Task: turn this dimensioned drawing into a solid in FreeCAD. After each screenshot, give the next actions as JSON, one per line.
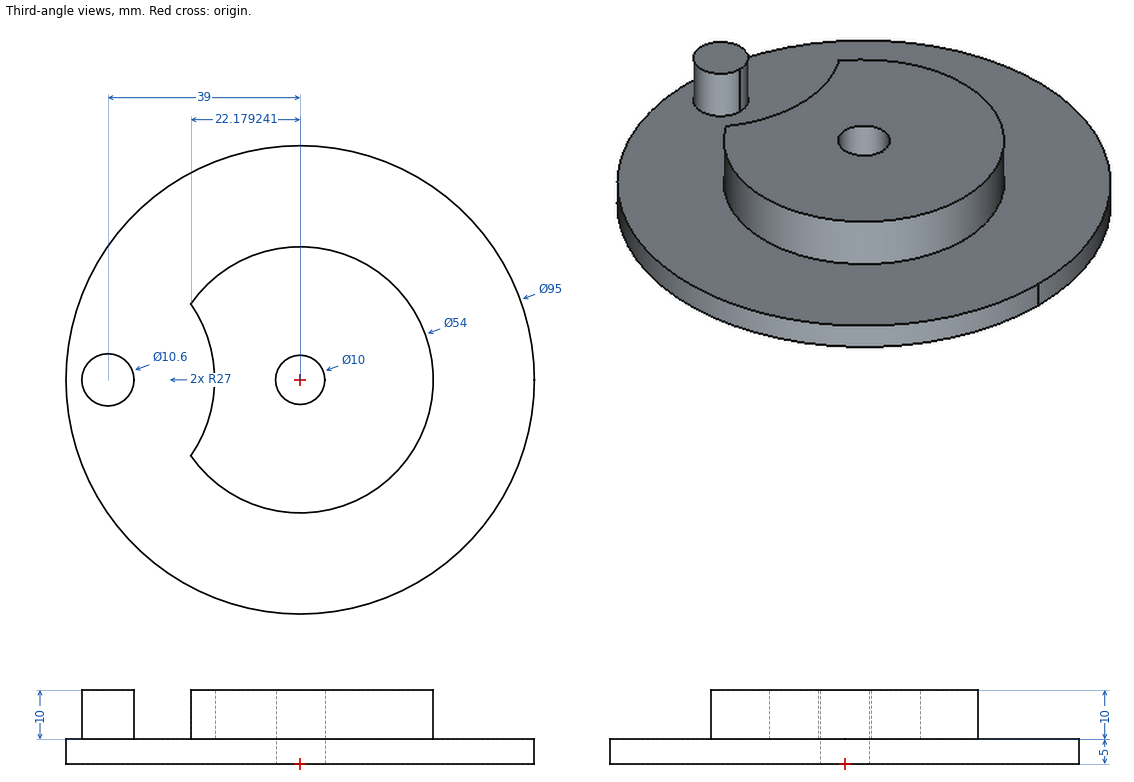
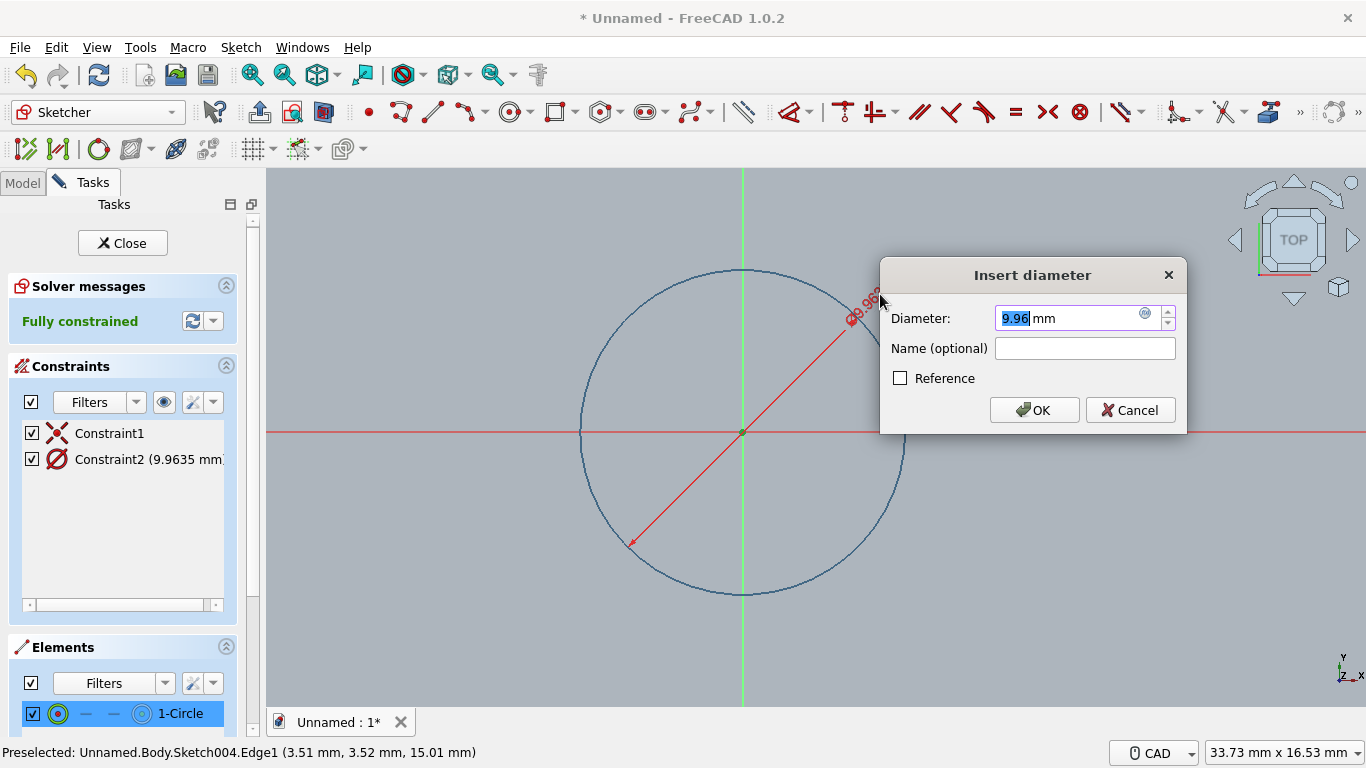
{"action": "type", "text": "10"}
{"action": "key", "text": "Return"}
{"action": "key", "text": "Escape"}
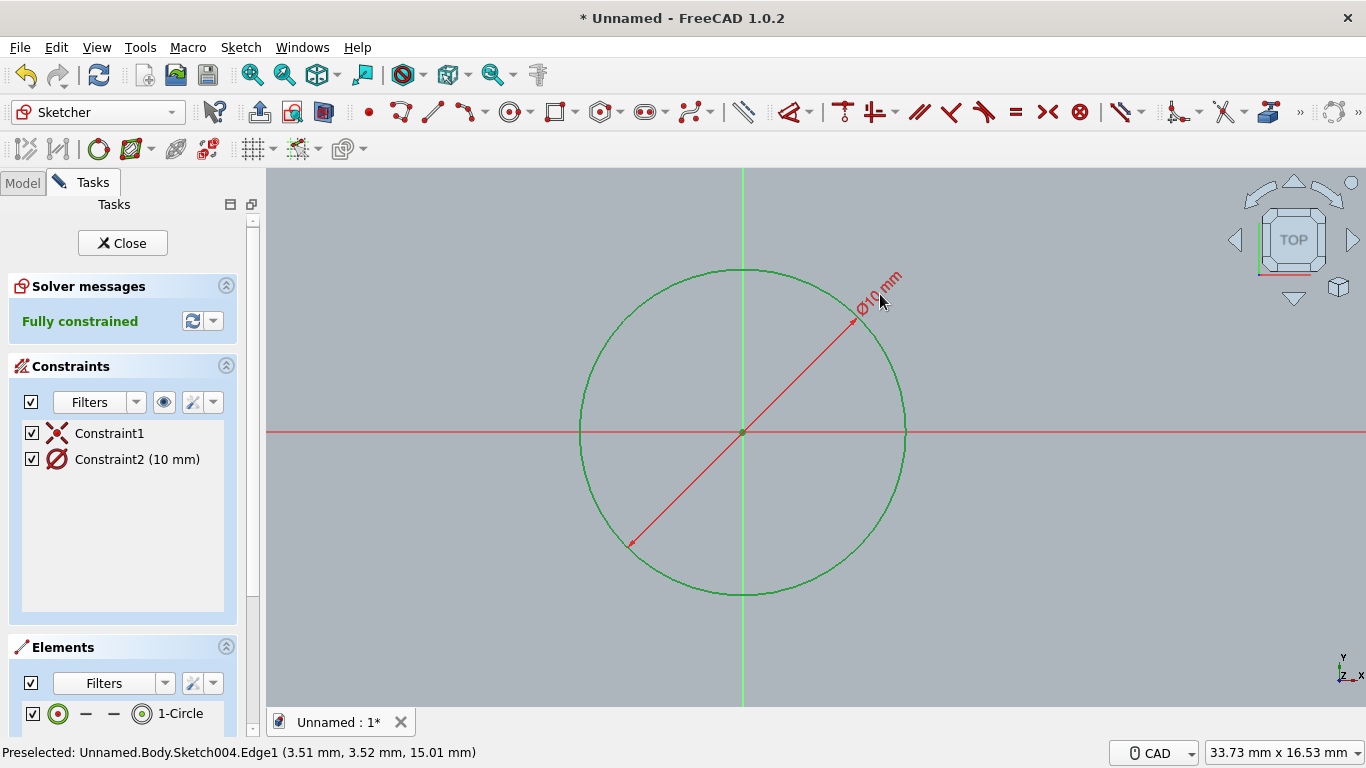
{"action": "left_click", "coordinate": [123, 243]}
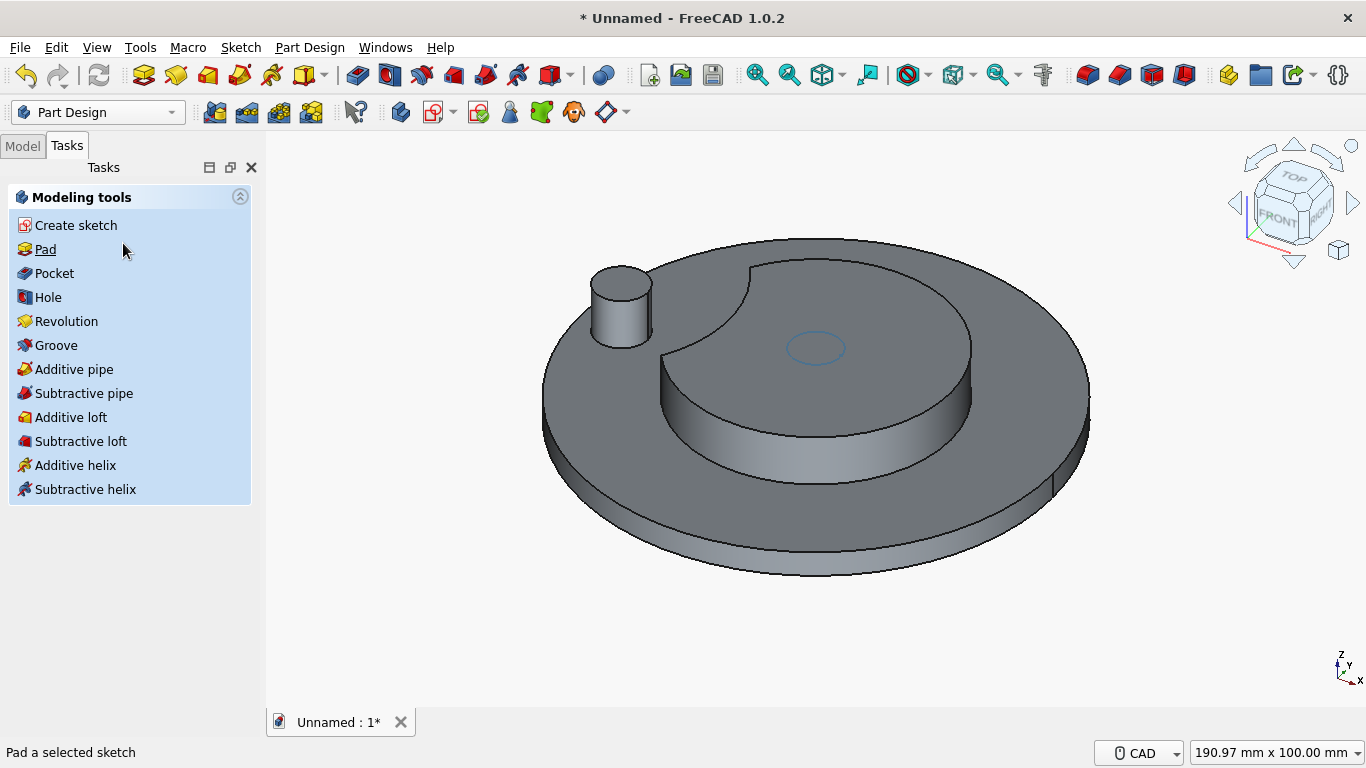
{"action": "left_click", "coordinate": [358, 76]}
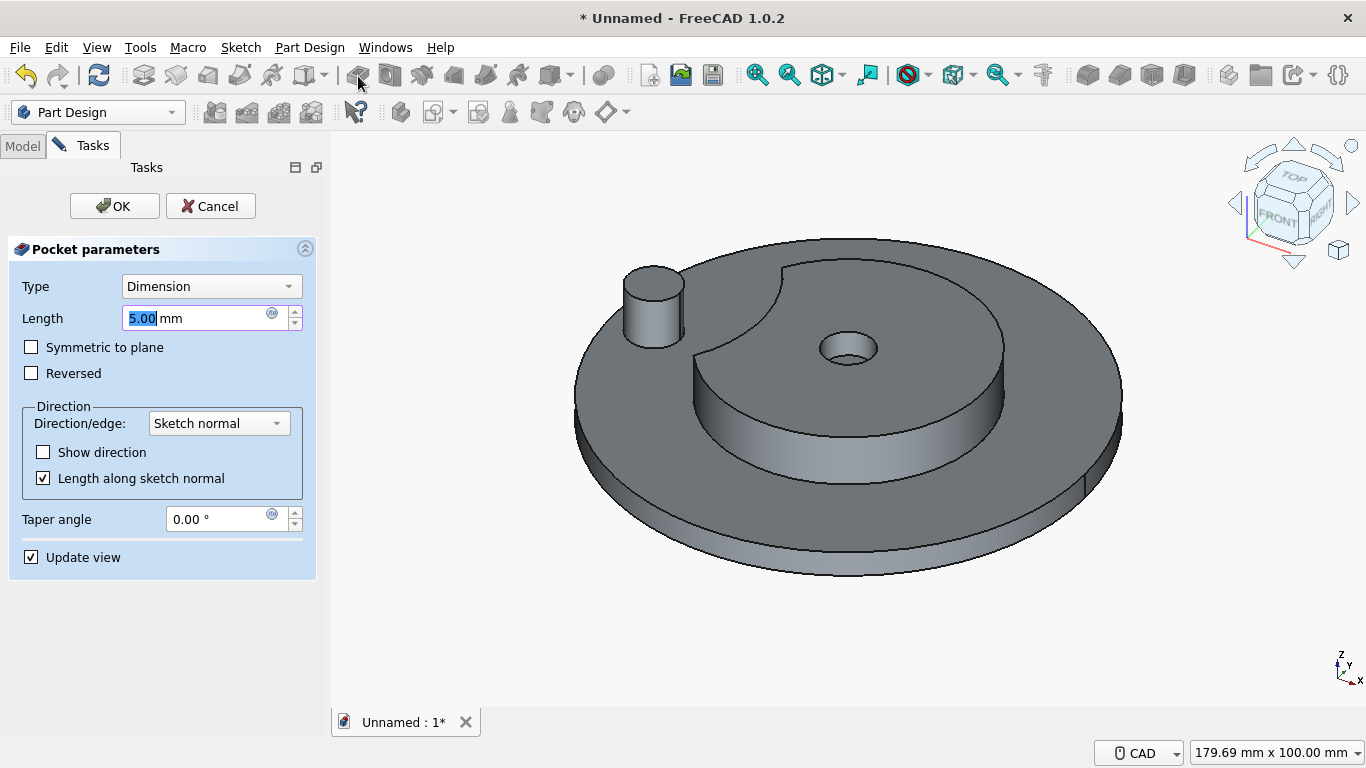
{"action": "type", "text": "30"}
{"action": "key", "text": "Tab"}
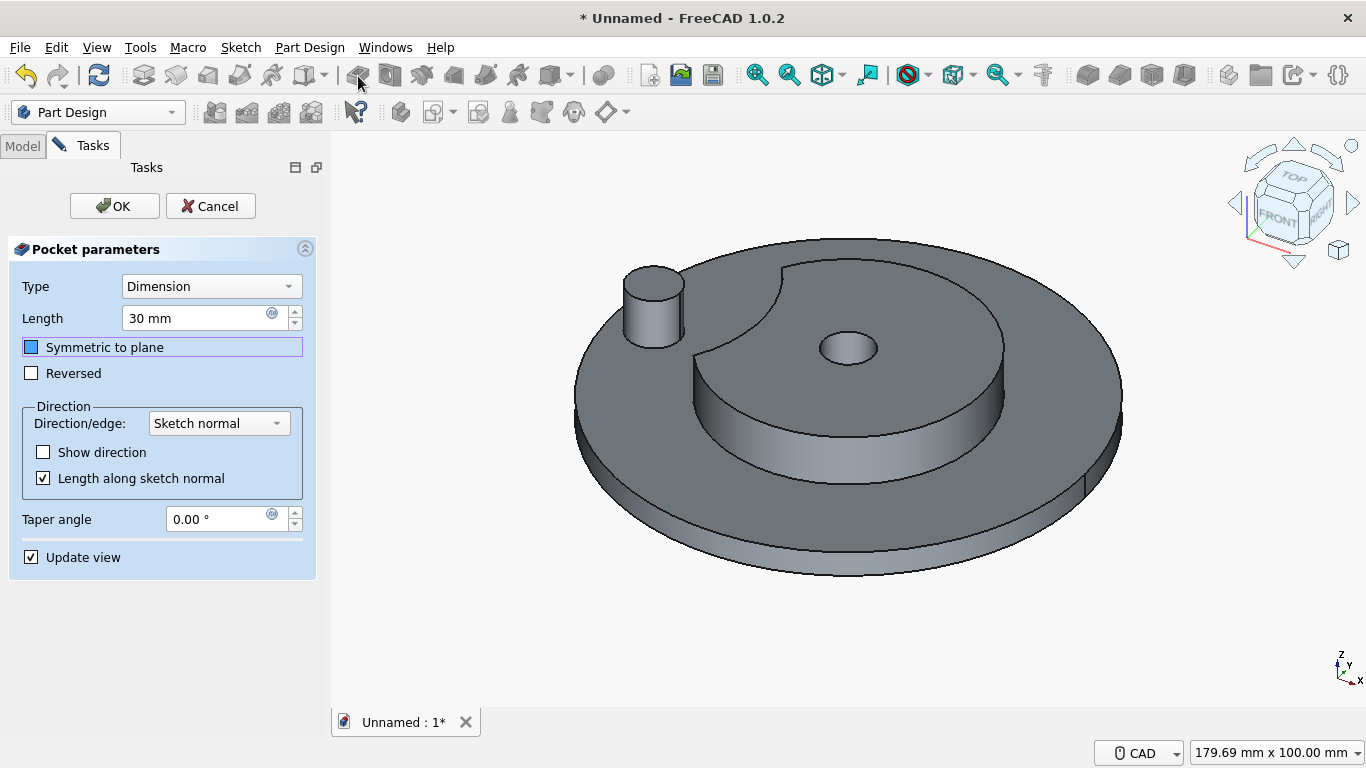
{"action": "left_click", "coordinate": [115, 206]}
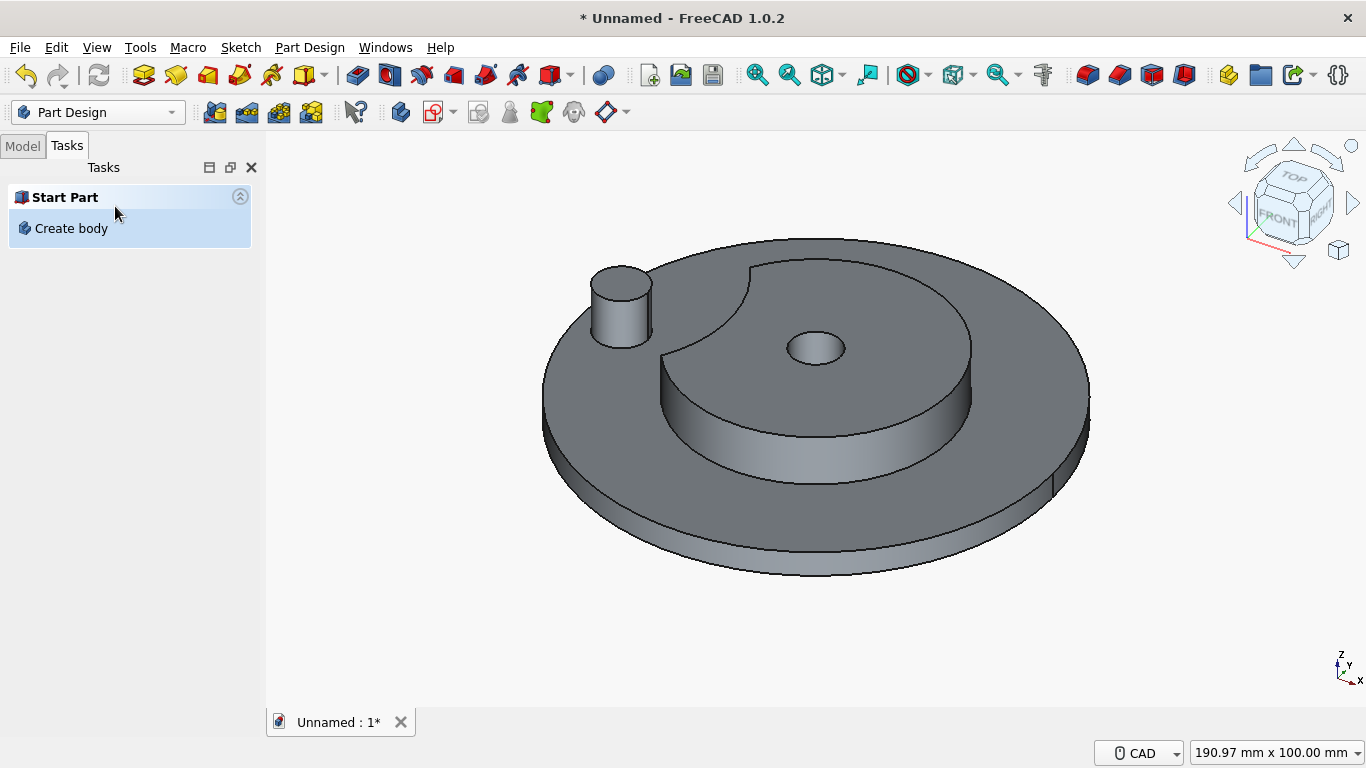
{"action": "key", "text": "0"}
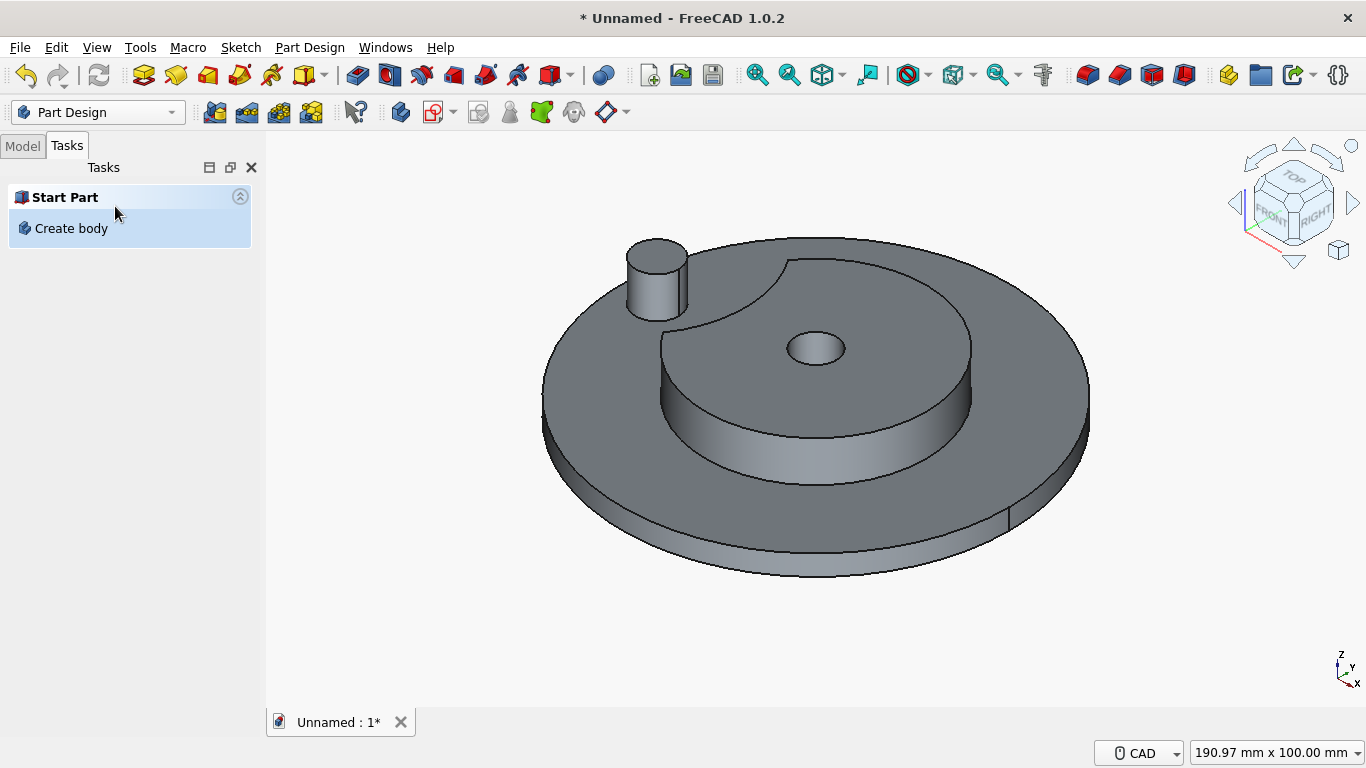
{"action": "key", "text": "v f"}